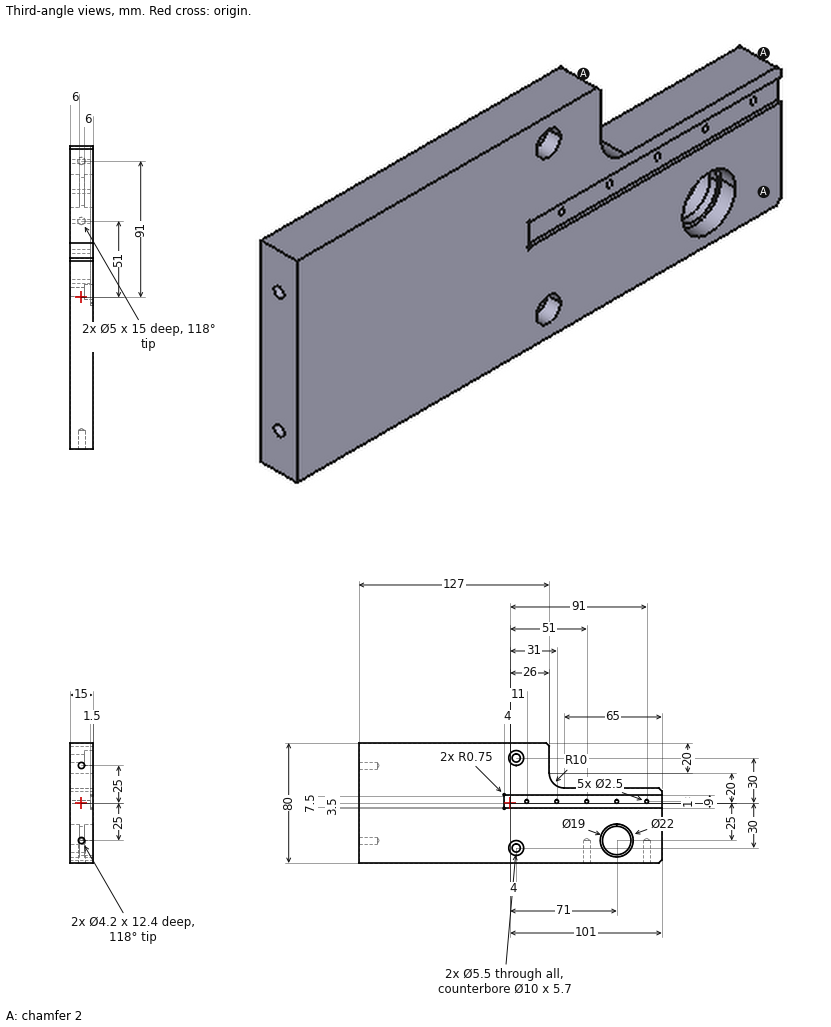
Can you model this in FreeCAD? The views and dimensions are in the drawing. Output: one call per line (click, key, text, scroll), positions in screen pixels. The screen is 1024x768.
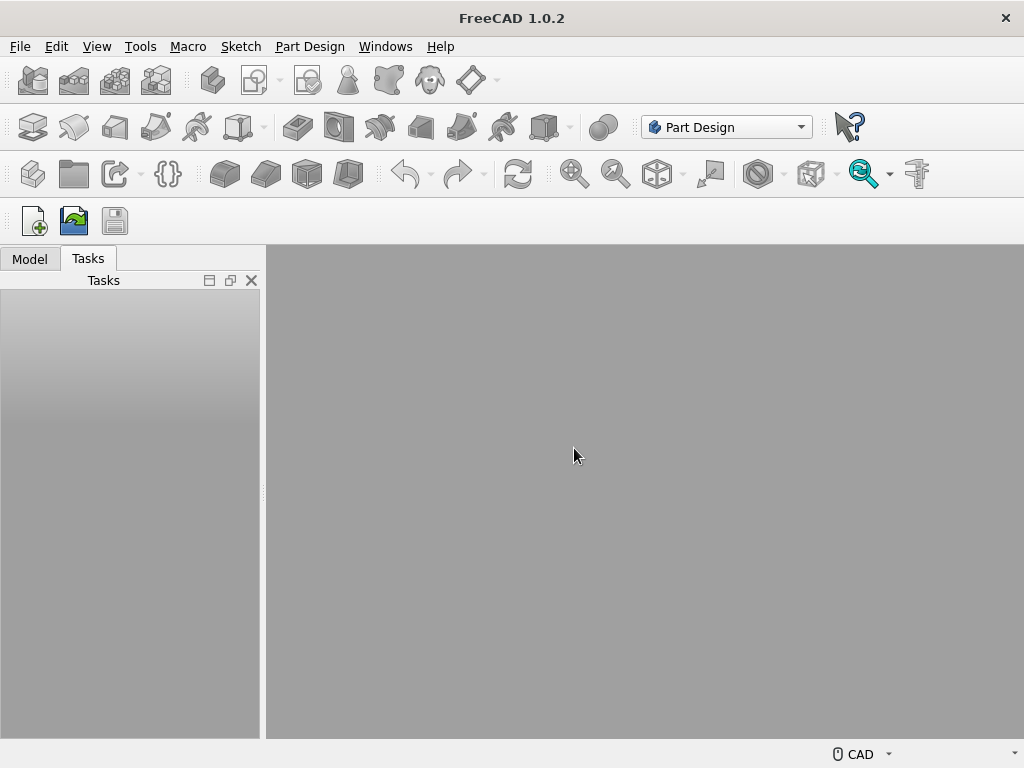
click(33, 222)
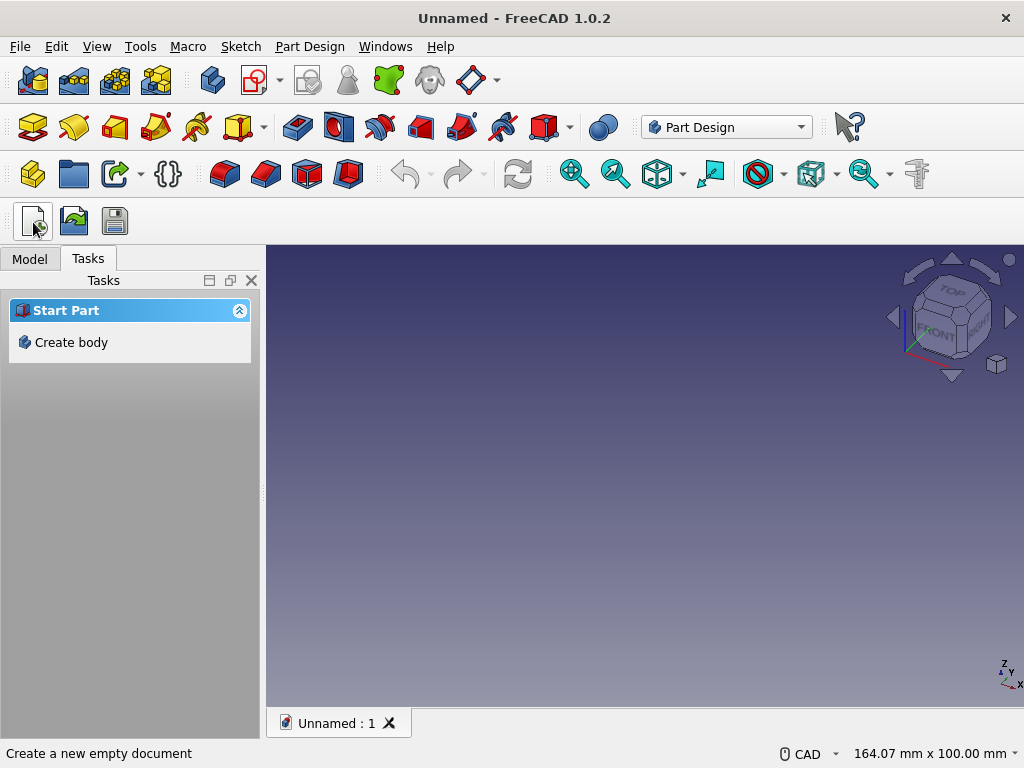
click(254, 80)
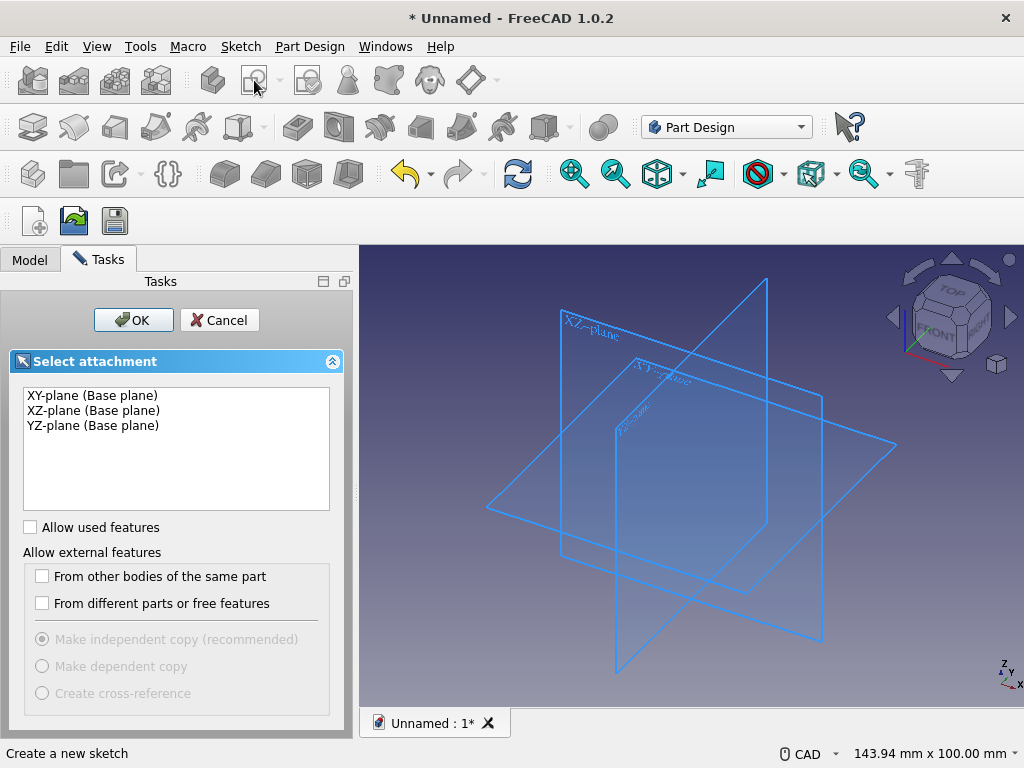
click(84, 426)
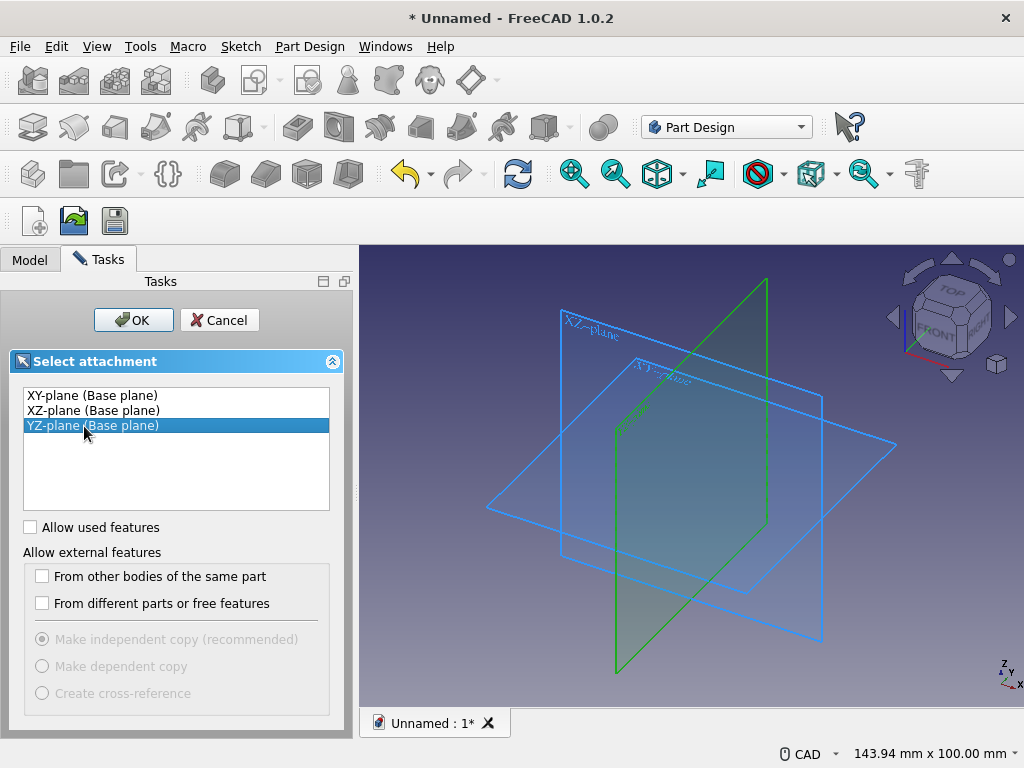
click(134, 320)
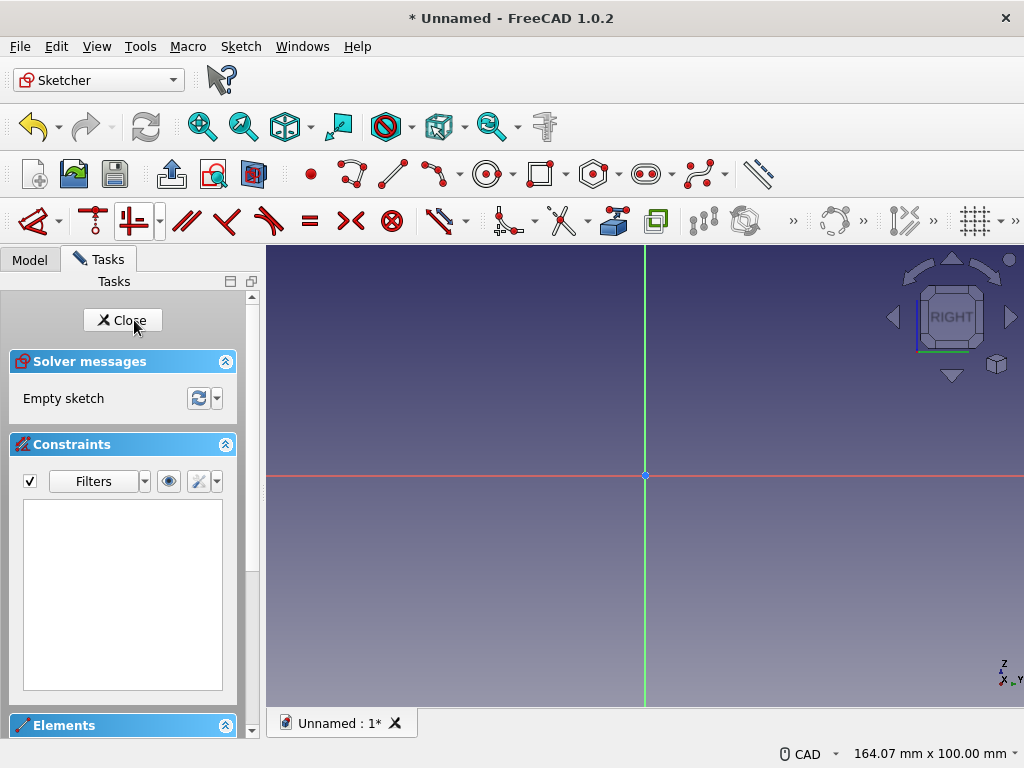
scroll(521, 476, down, 4)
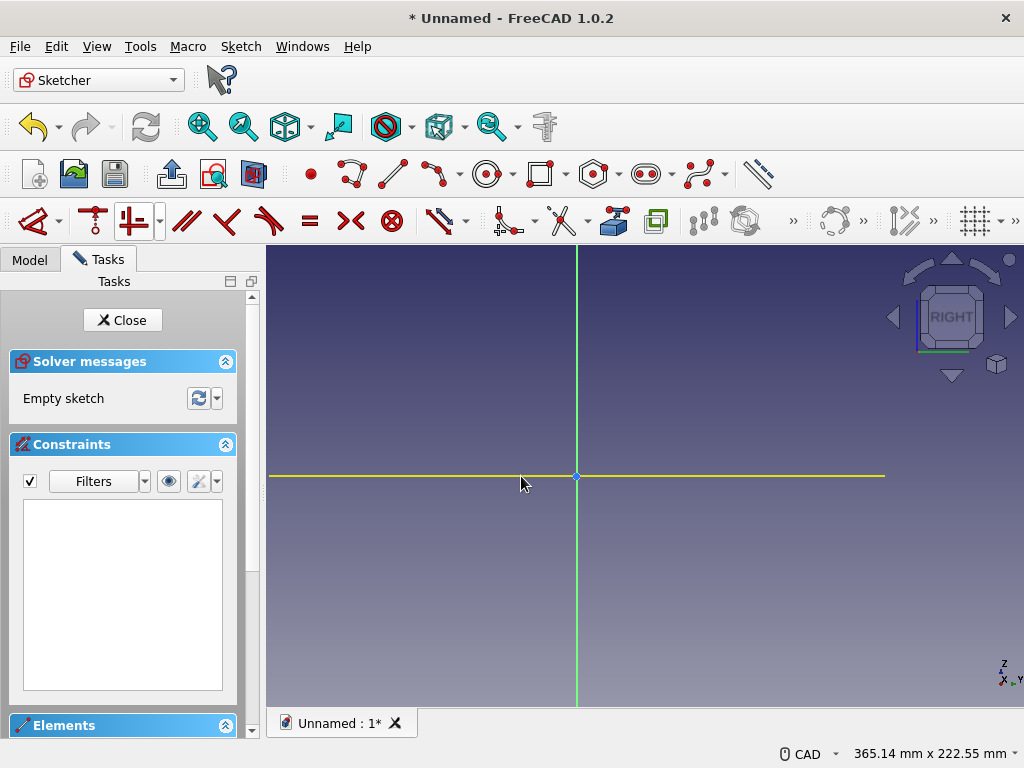
click(352, 174)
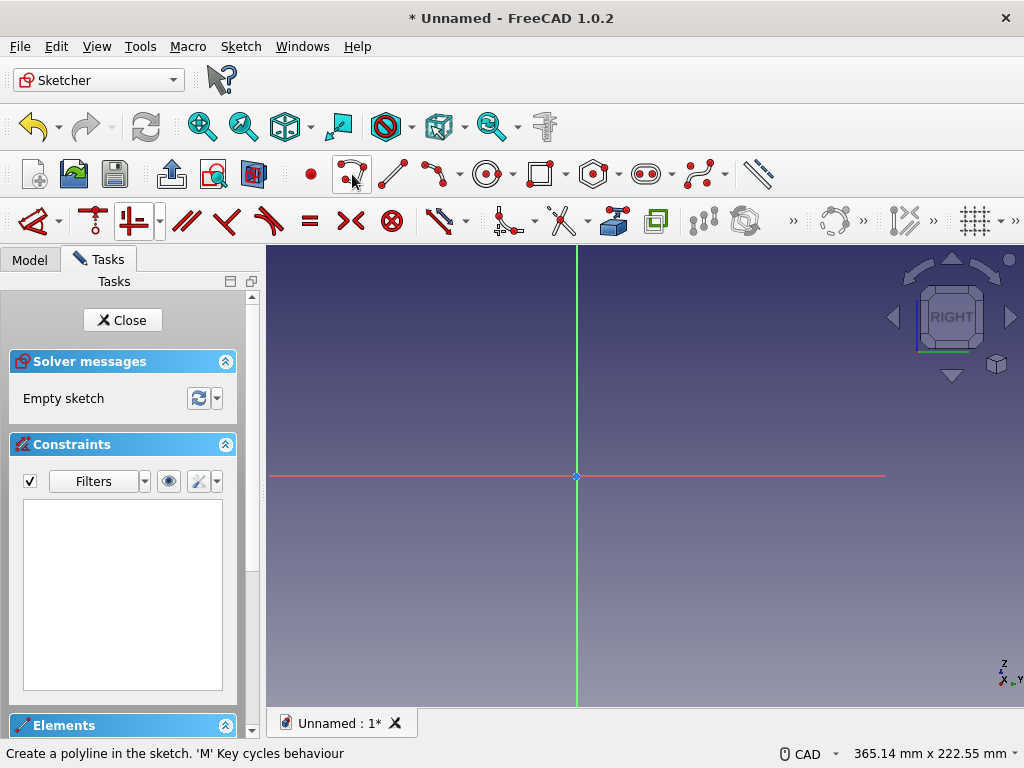
click(631, 435)
click(631, 393)
click(367, 393)
click(367, 559)
click(787, 559)
click(787, 456)
click(652, 456)
right_click(652, 456)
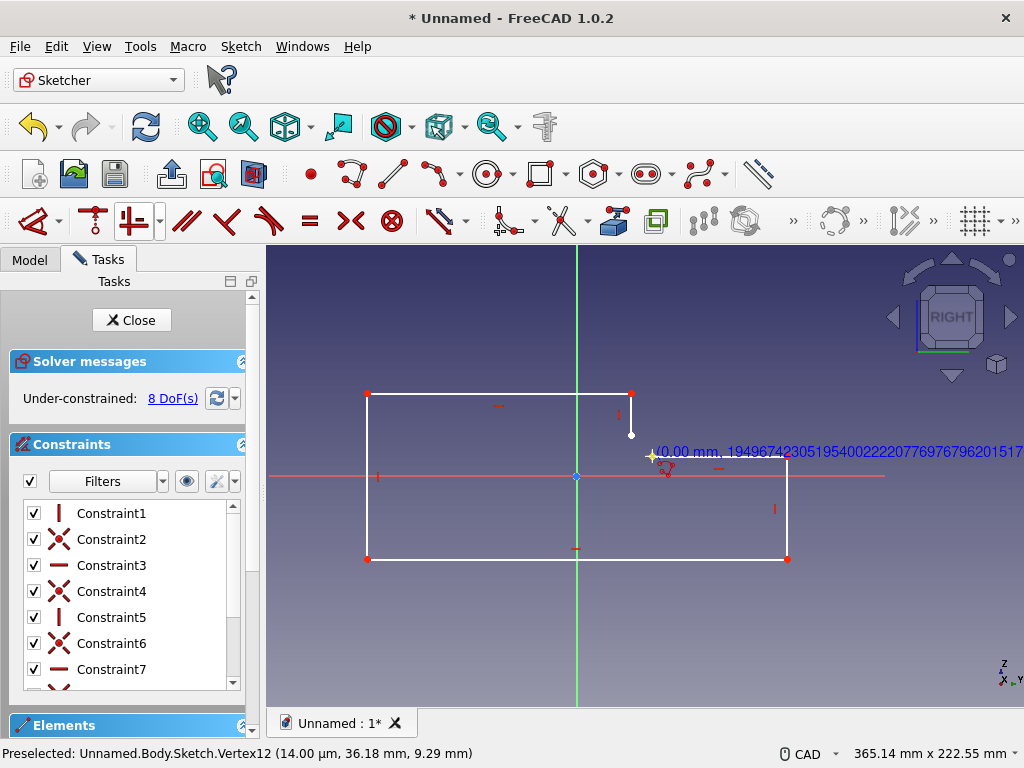
click(434, 174)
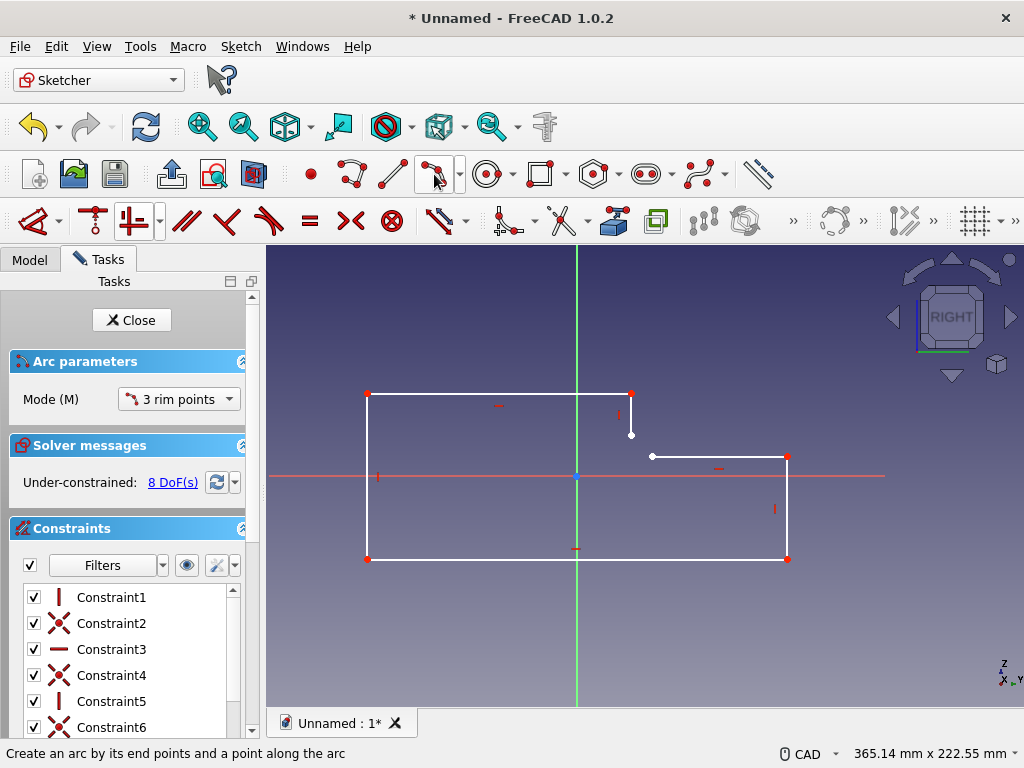
click(652, 457)
click(631, 436)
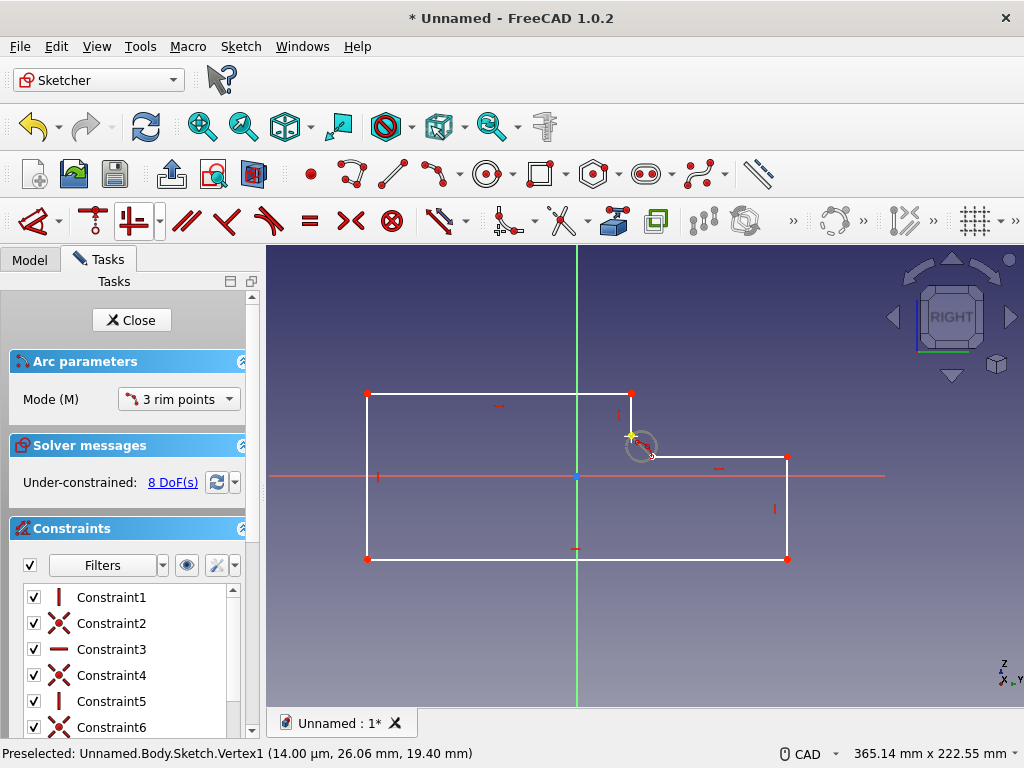
scroll(637, 449, up, 5)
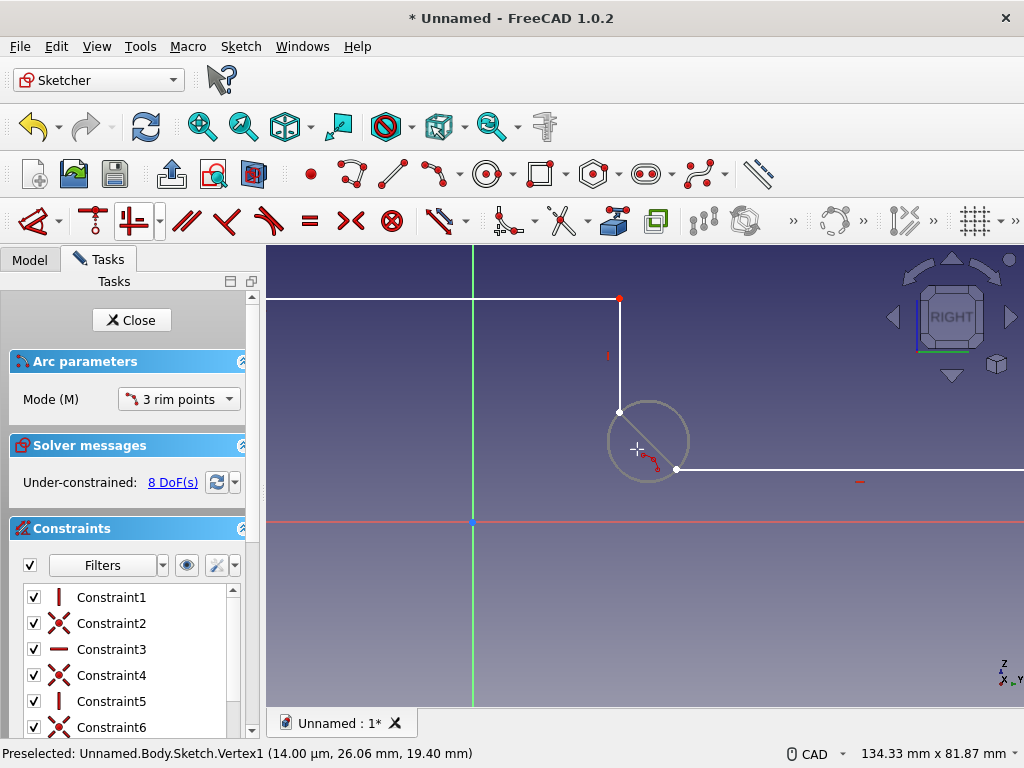
click(636, 449)
key(Escape)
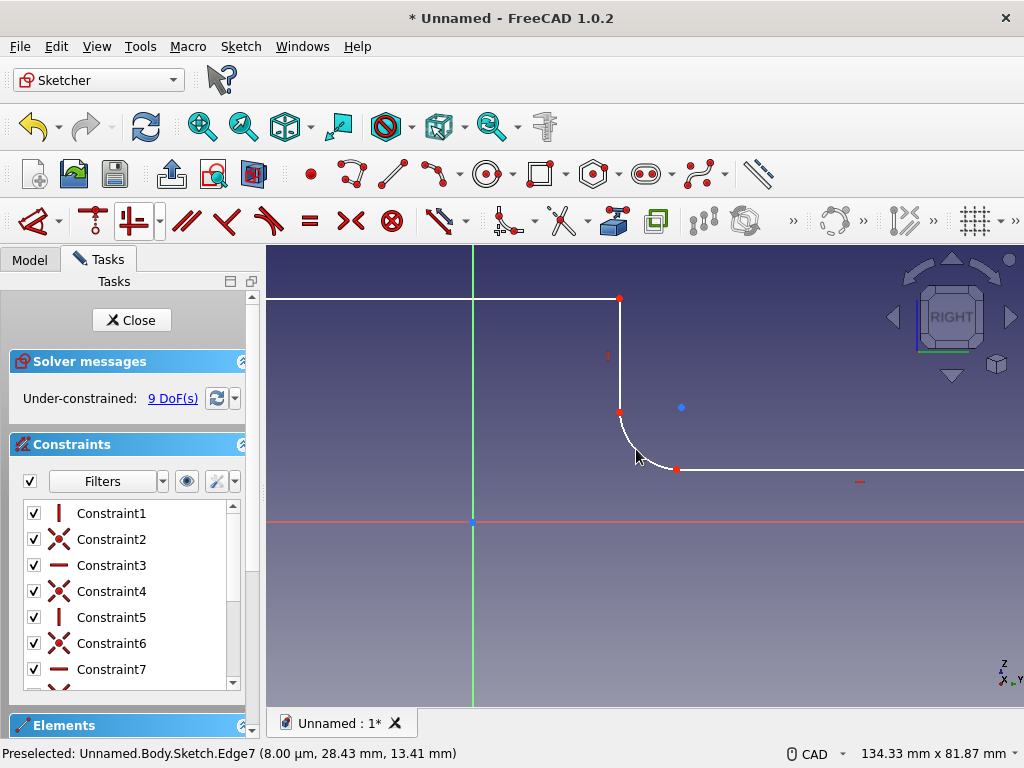
click(620, 379)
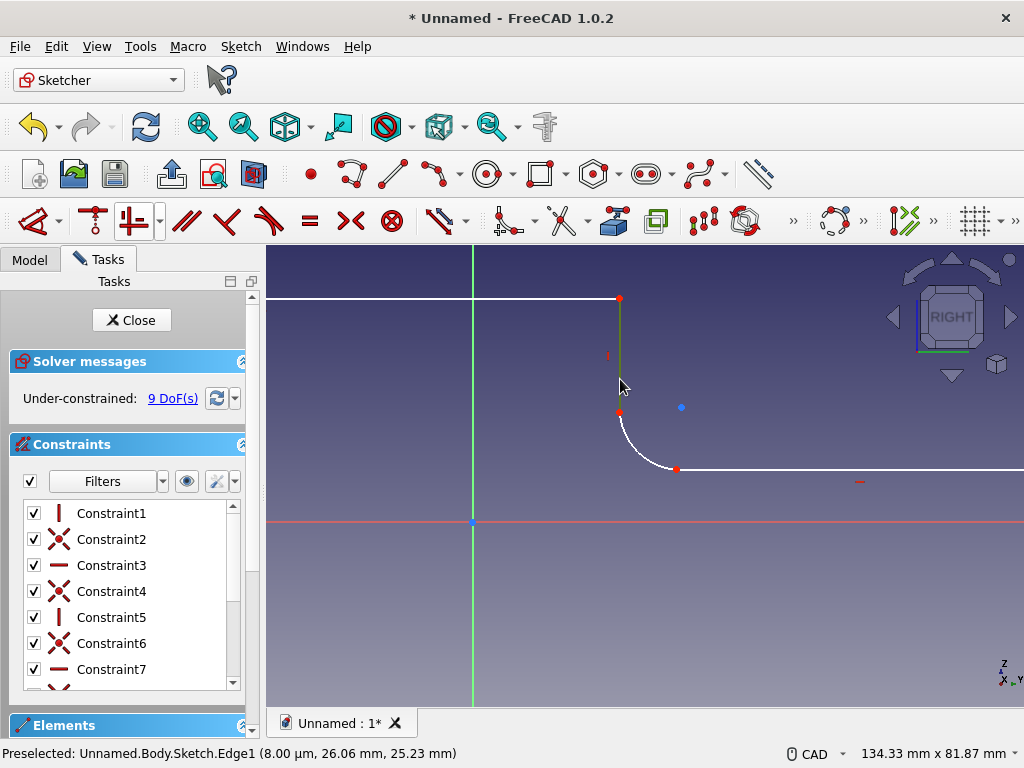
click(627, 438)